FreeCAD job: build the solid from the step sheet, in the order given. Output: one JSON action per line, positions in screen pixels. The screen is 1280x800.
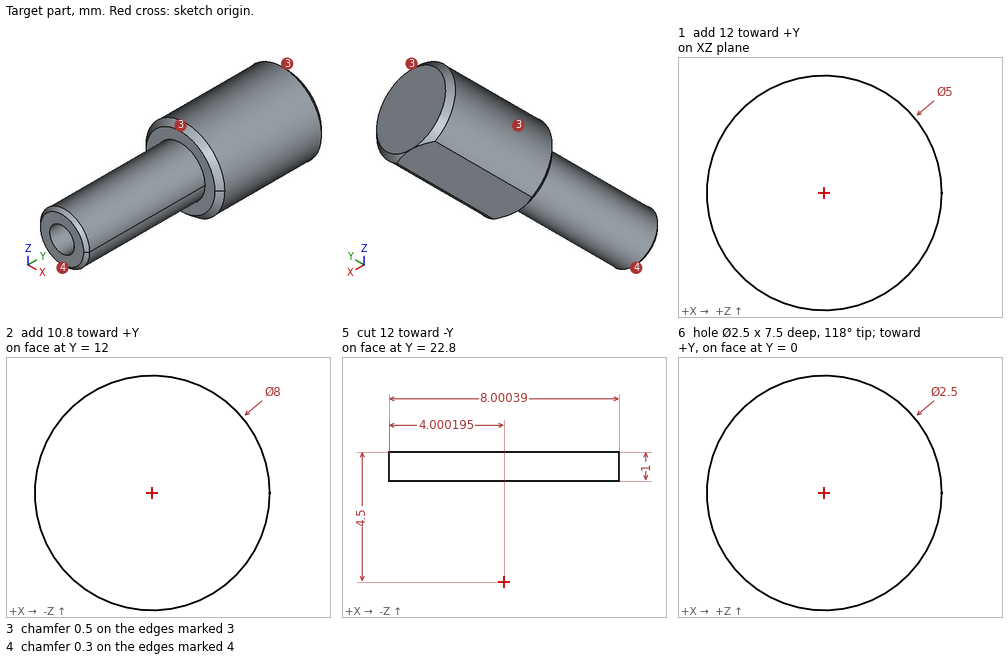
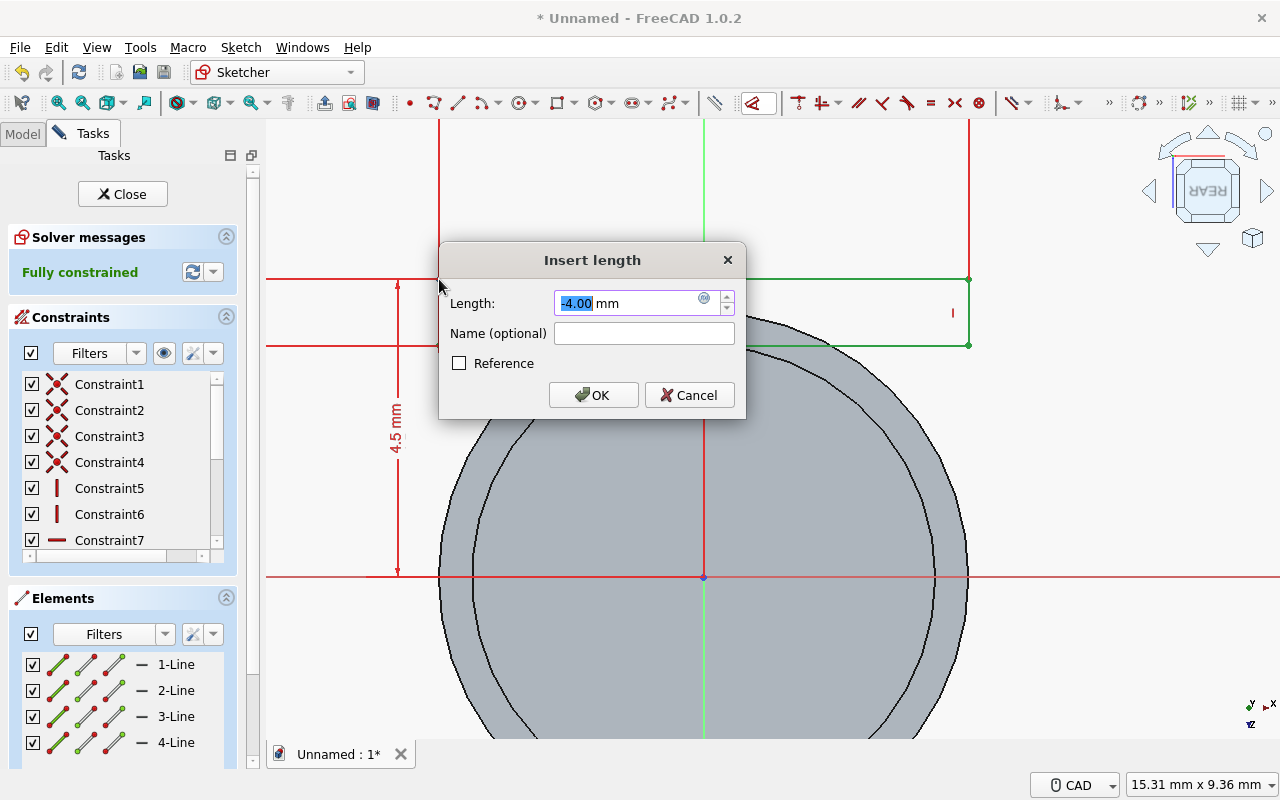
{"action": "type", "text": "-4.000195"}
{"action": "key", "text": "Return"}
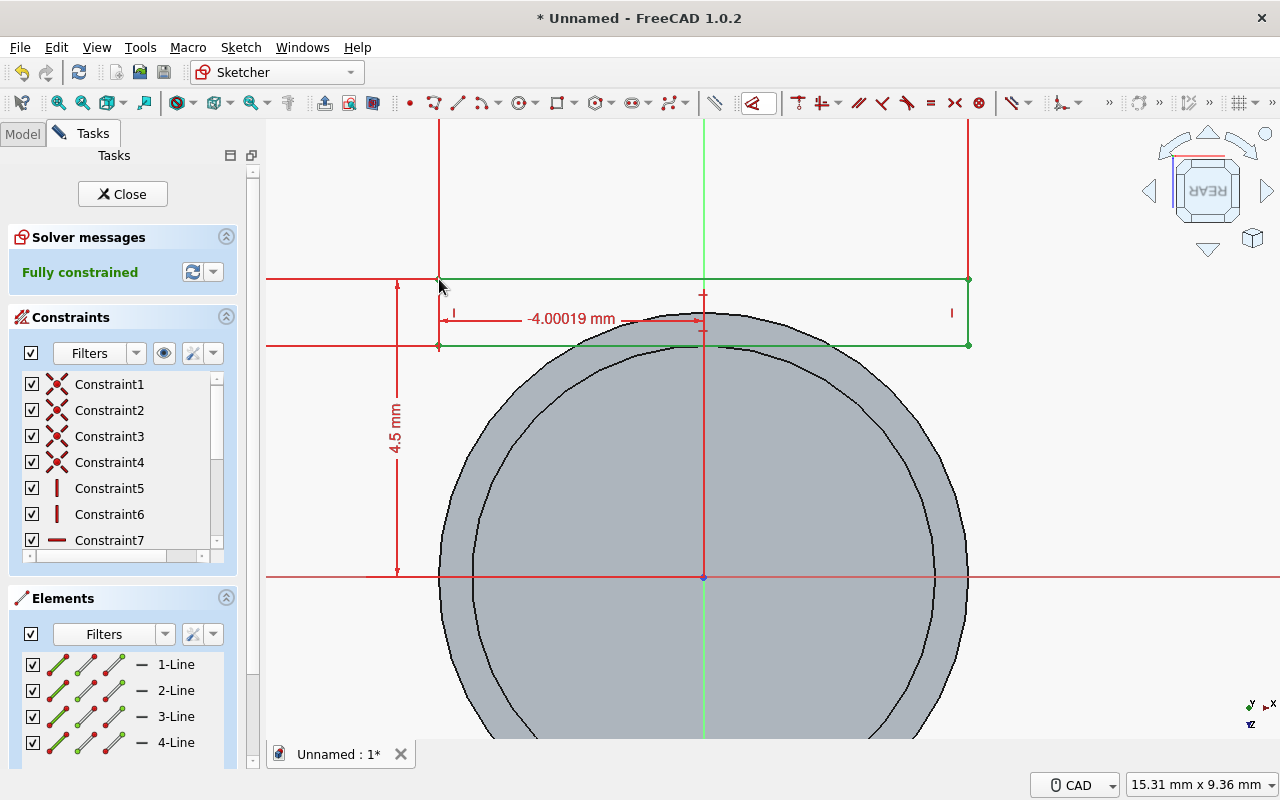
{"action": "left_click", "coordinate": [123, 194]}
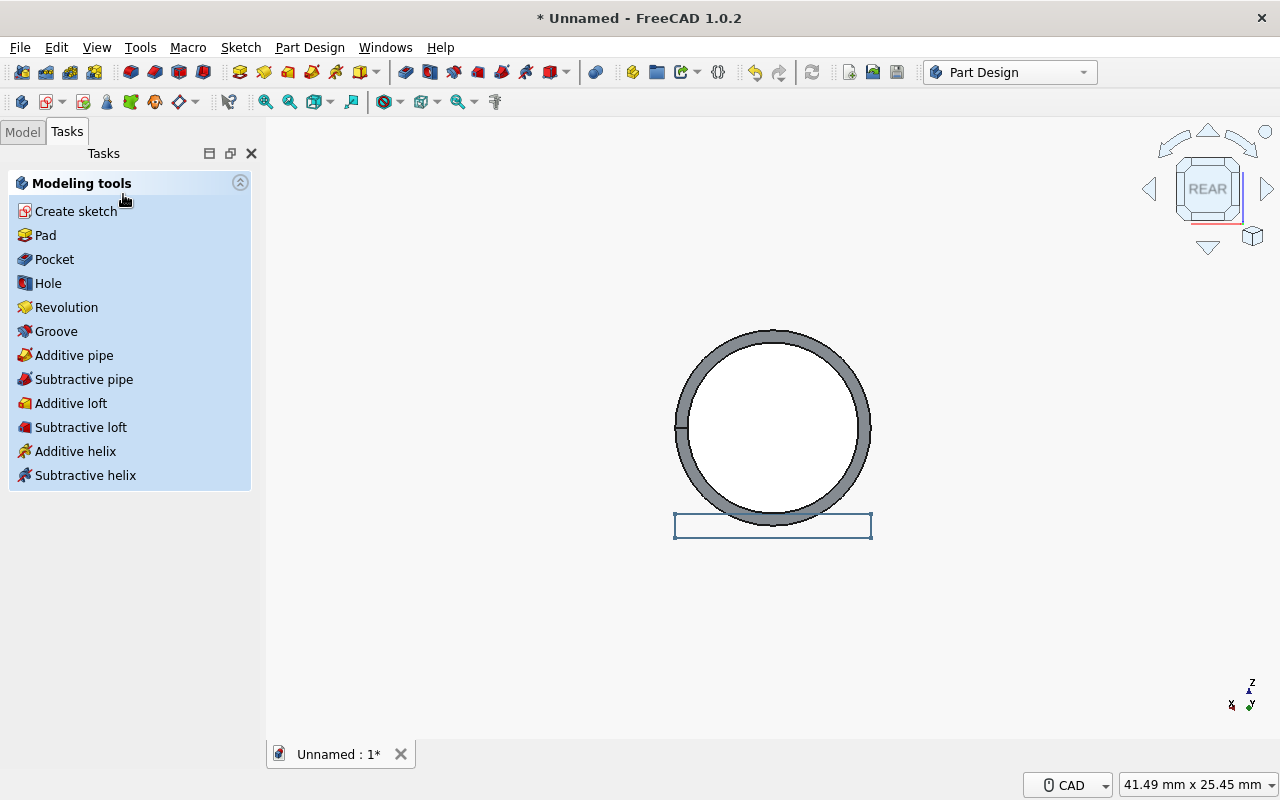
{"action": "left_click", "coordinate": [406, 72]}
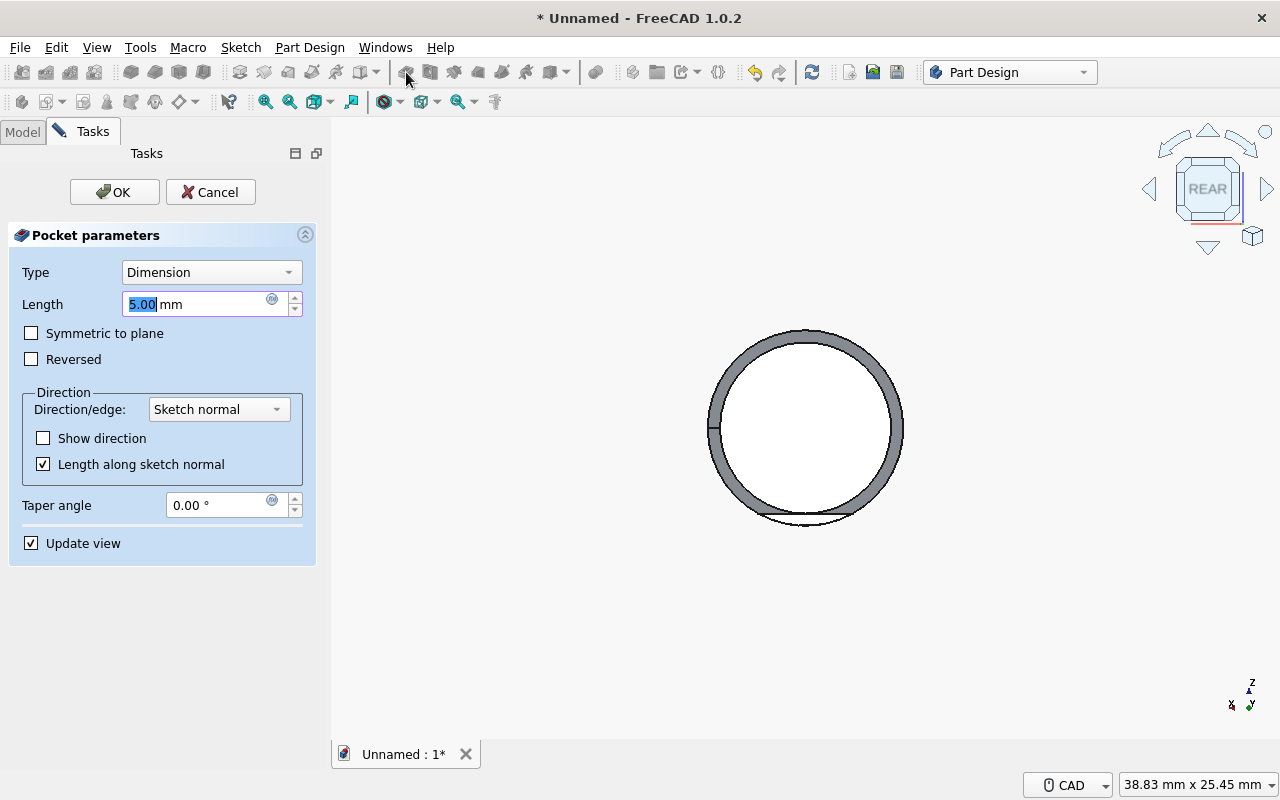
{"action": "type", "text": "12"}
{"action": "key", "text": "Tab"}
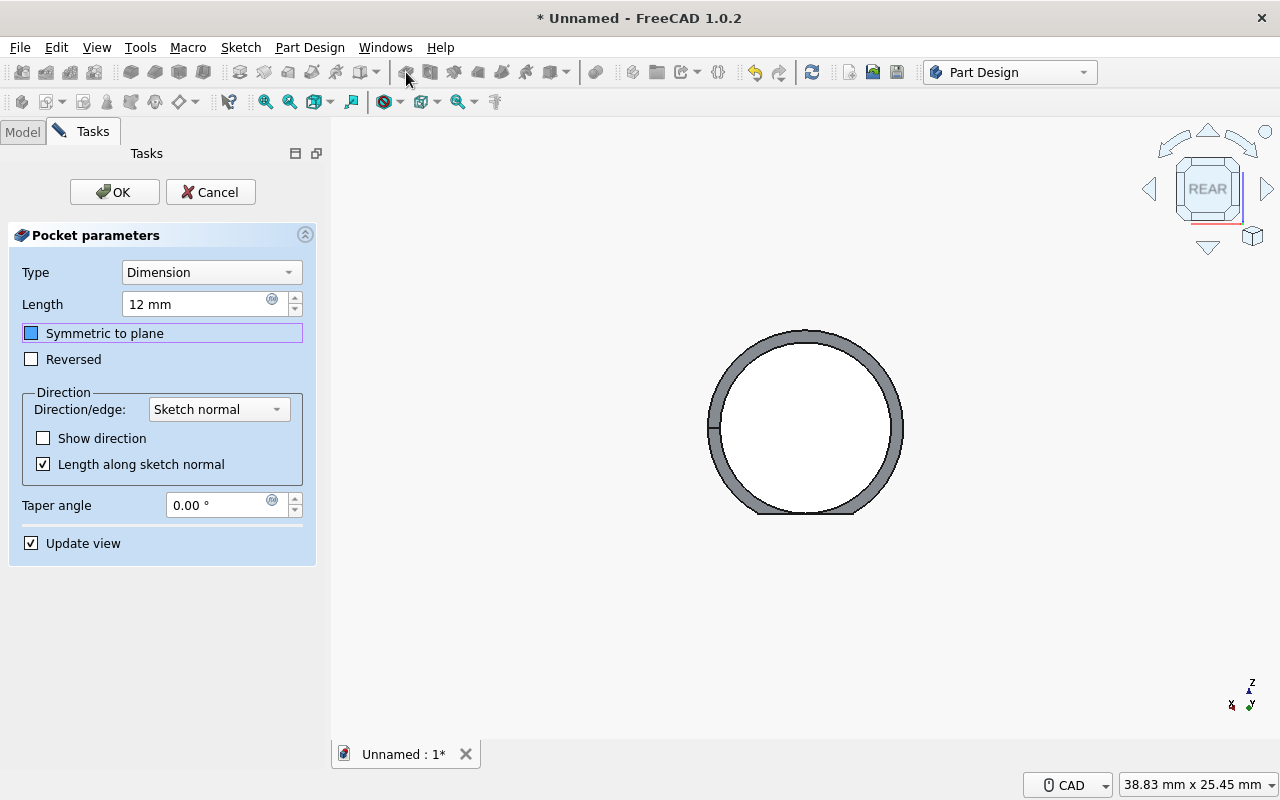
{"action": "left_click", "coordinate": [115, 192]}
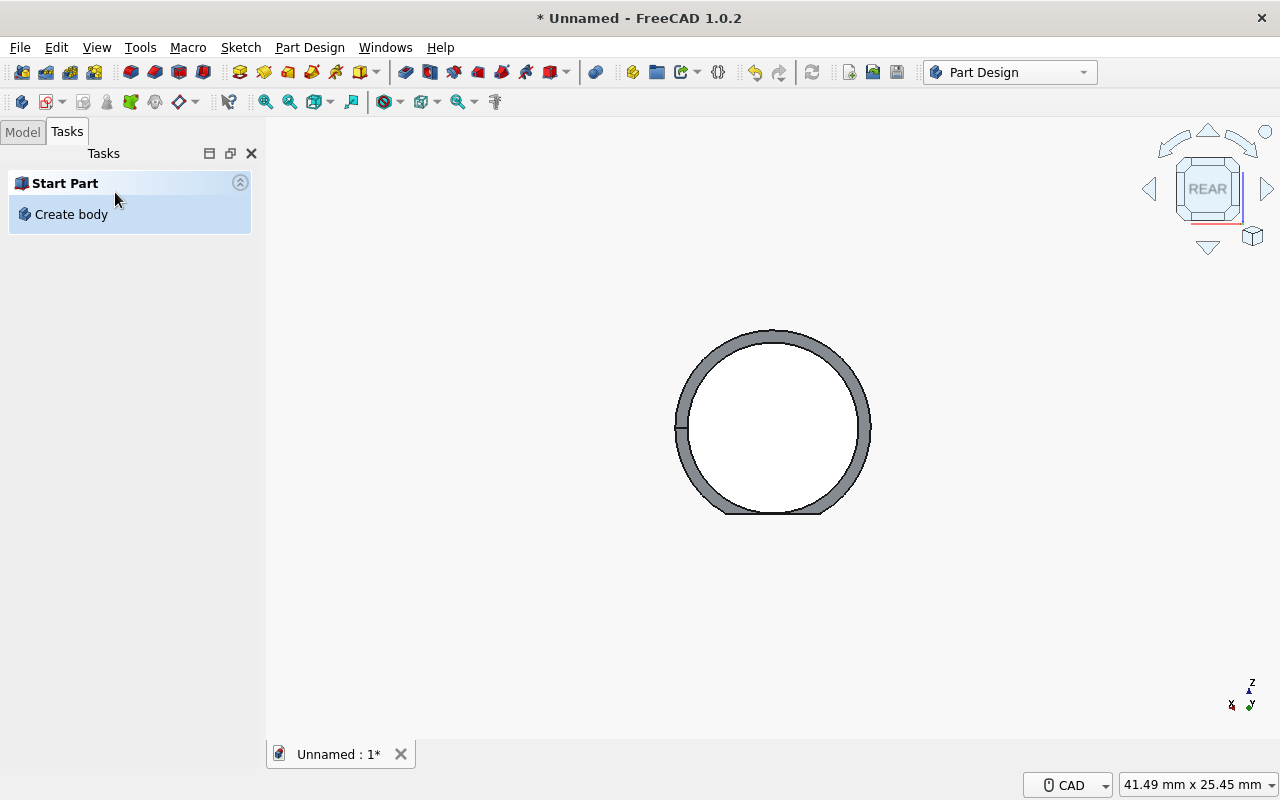
{"action": "key", "text": "v f"}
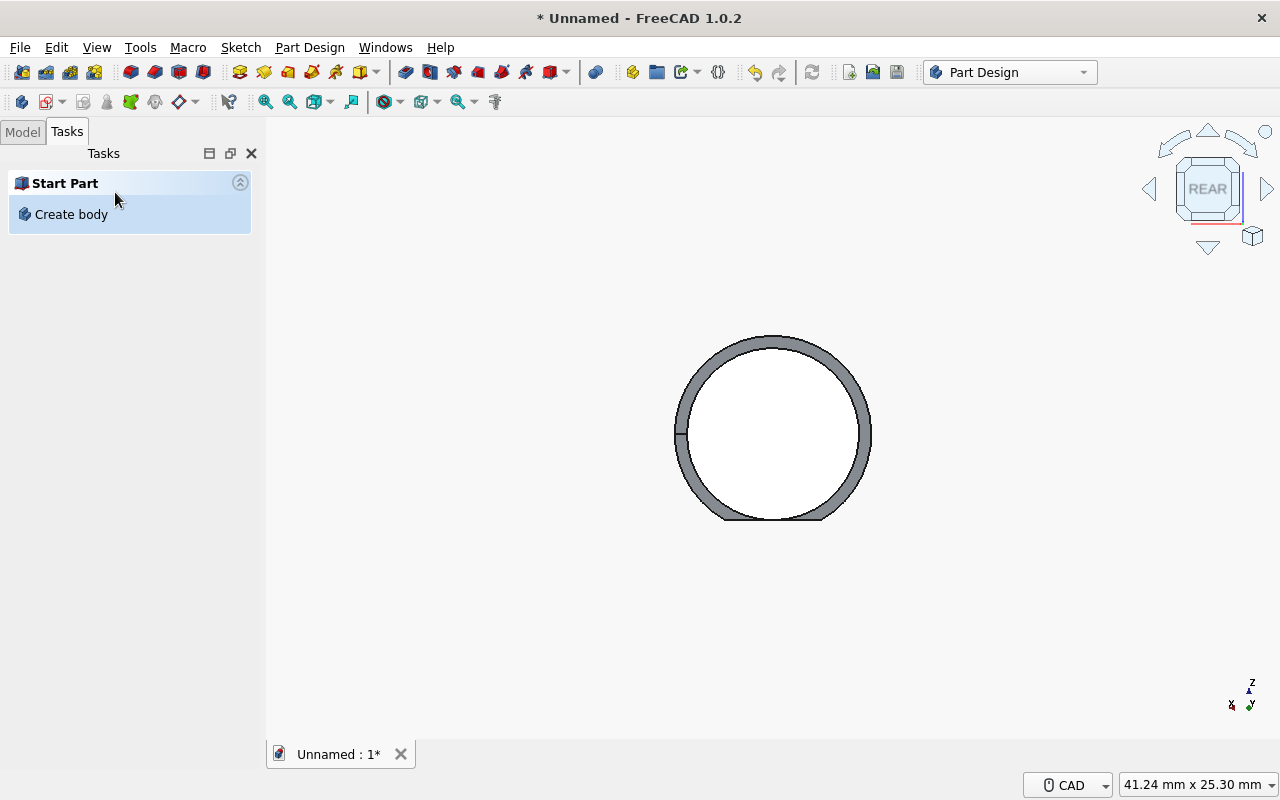
{"action": "key", "text": "0"}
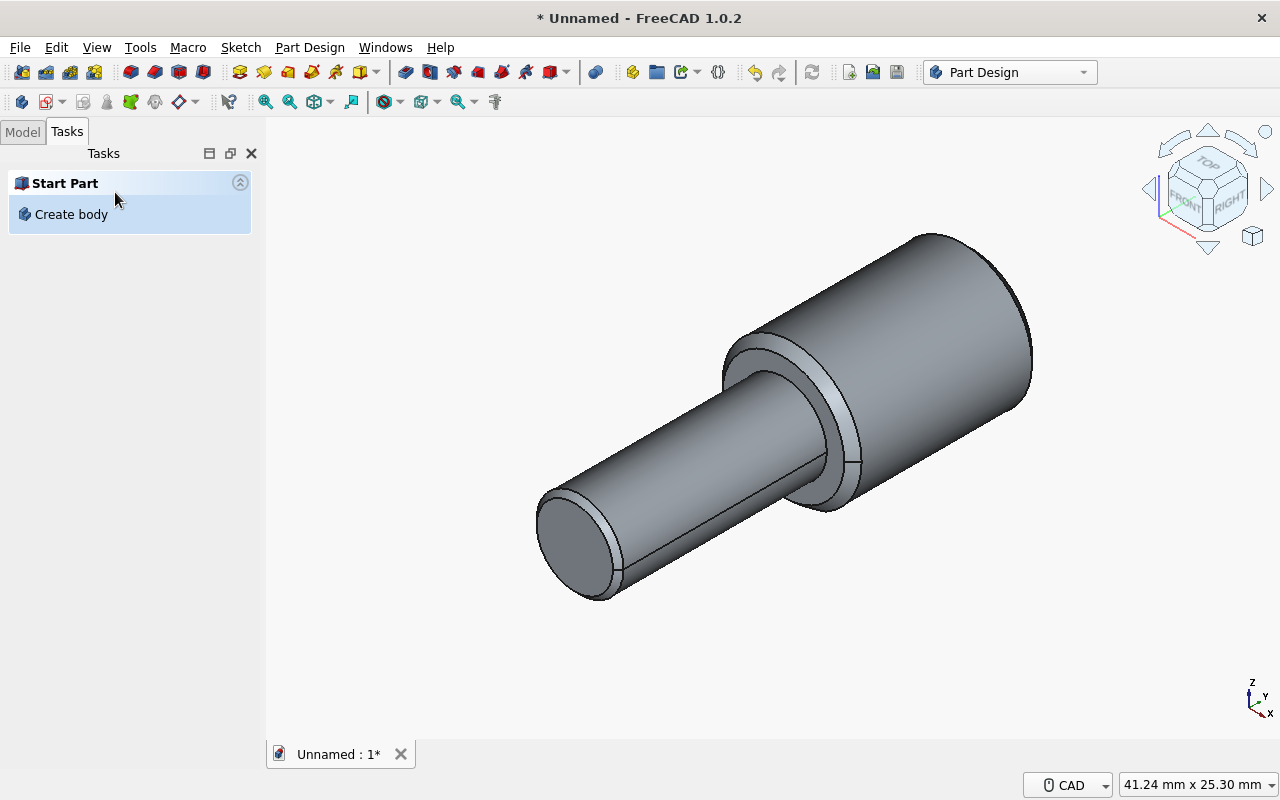
{"action": "left_click", "coordinate": [575, 546]}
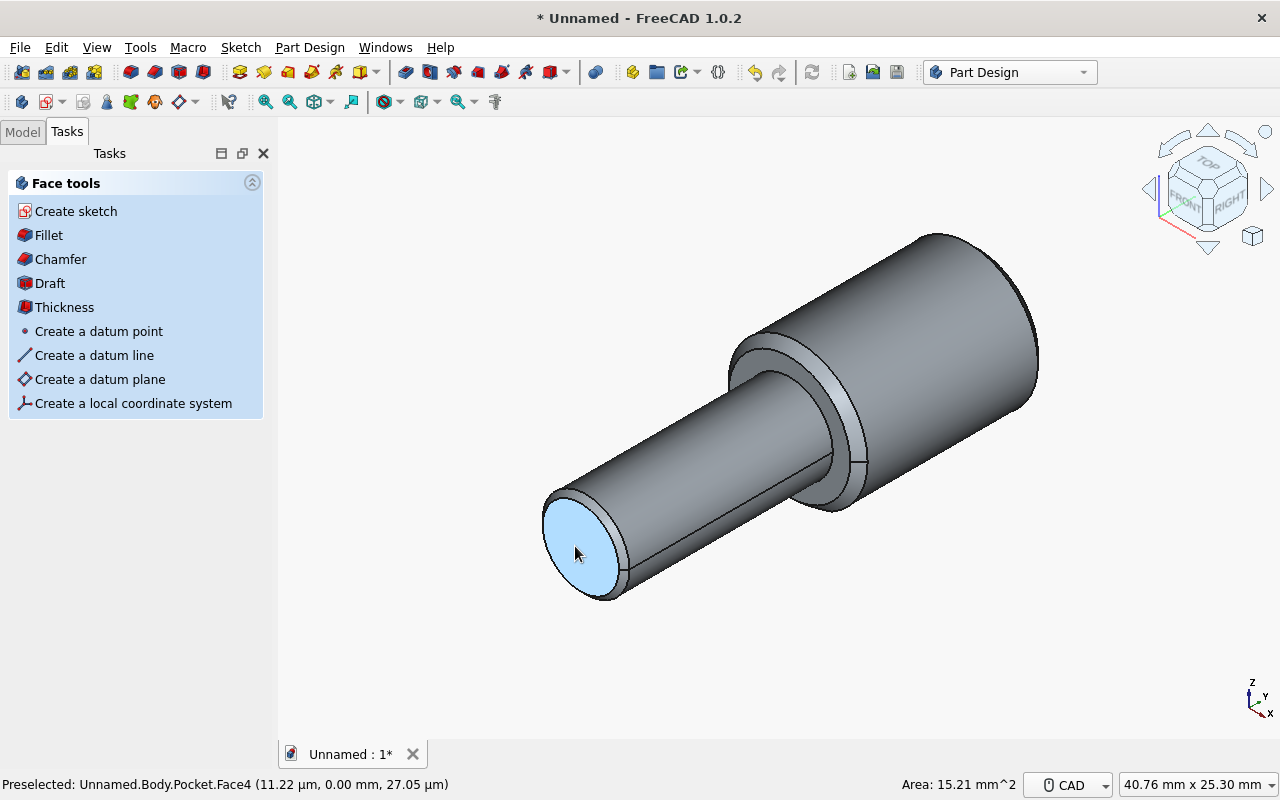
{"action": "left_click", "coordinate": [46, 102]}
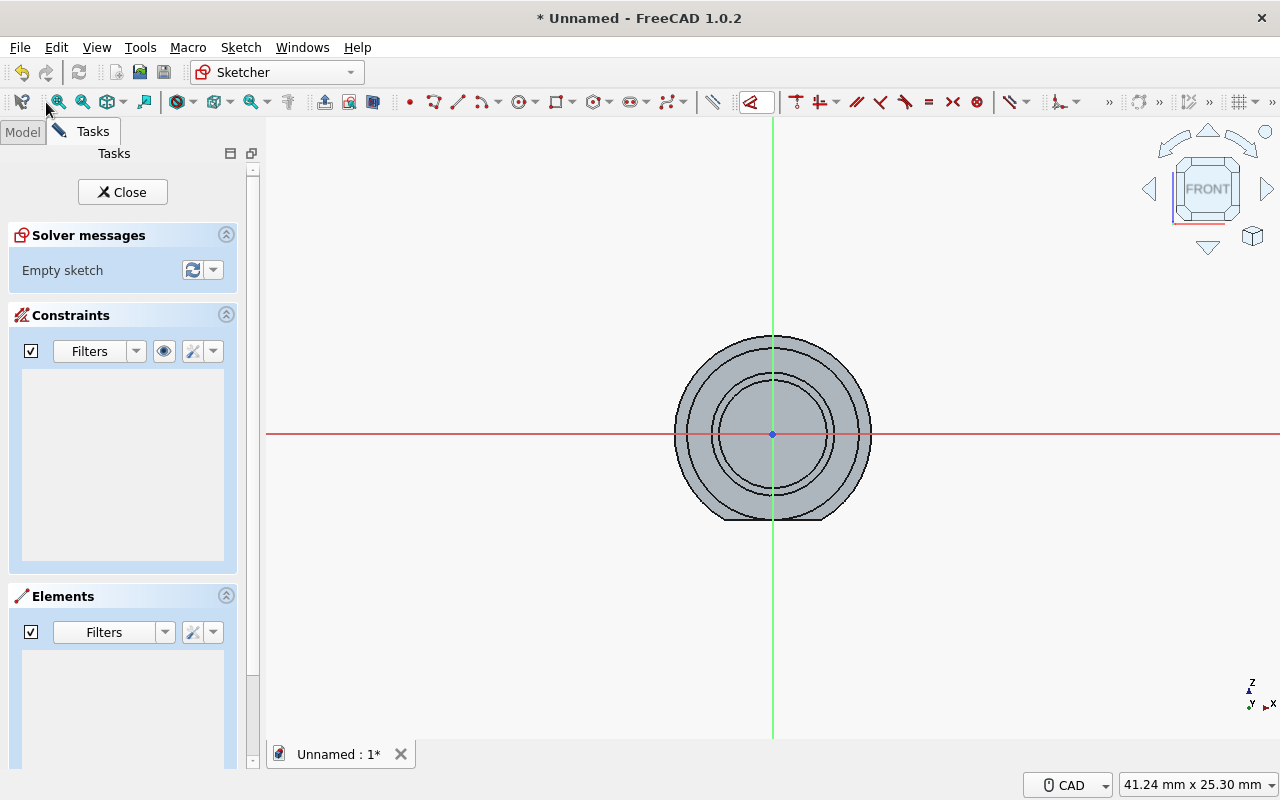
{"action": "scroll", "coordinate": [787, 435], "scroll_direction": "up", "scroll_amount": 9}